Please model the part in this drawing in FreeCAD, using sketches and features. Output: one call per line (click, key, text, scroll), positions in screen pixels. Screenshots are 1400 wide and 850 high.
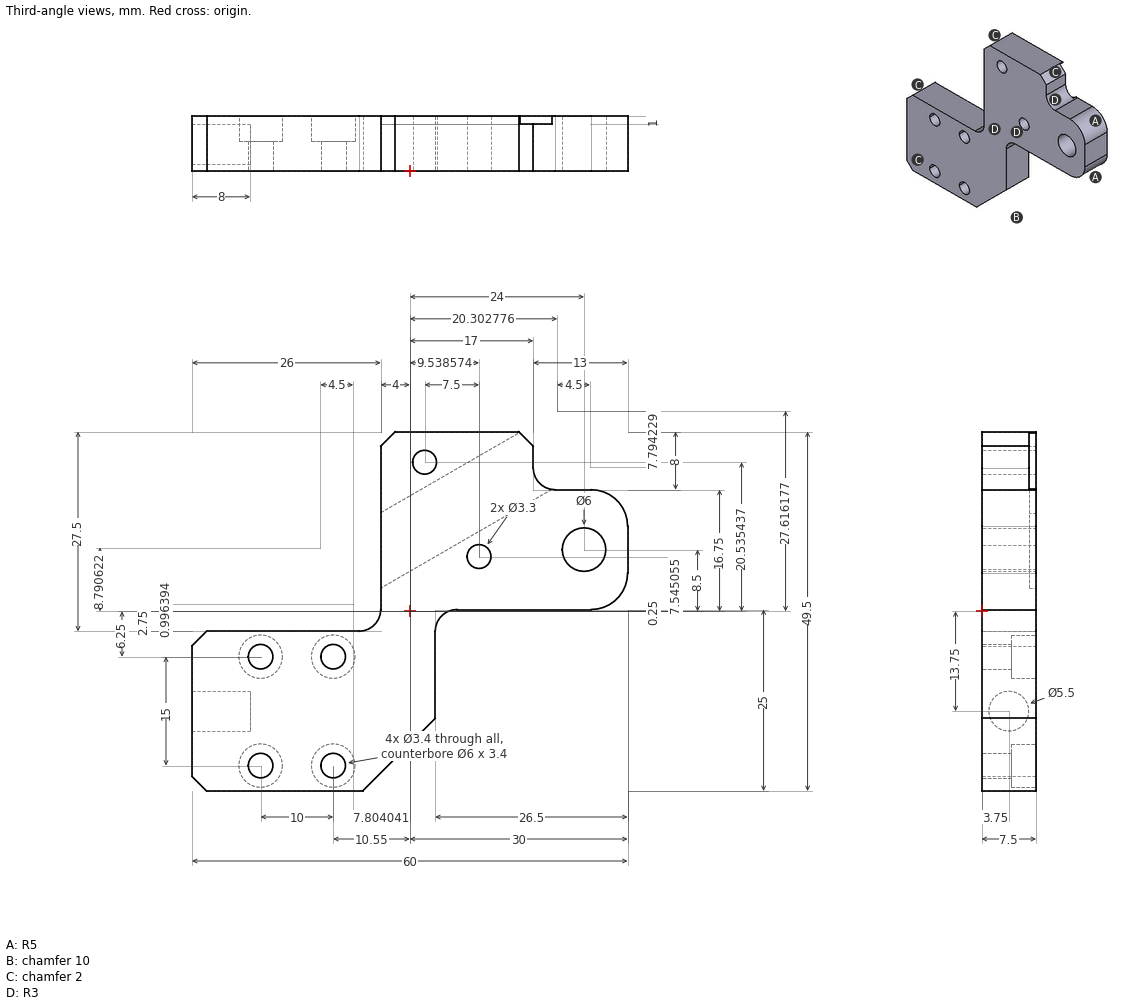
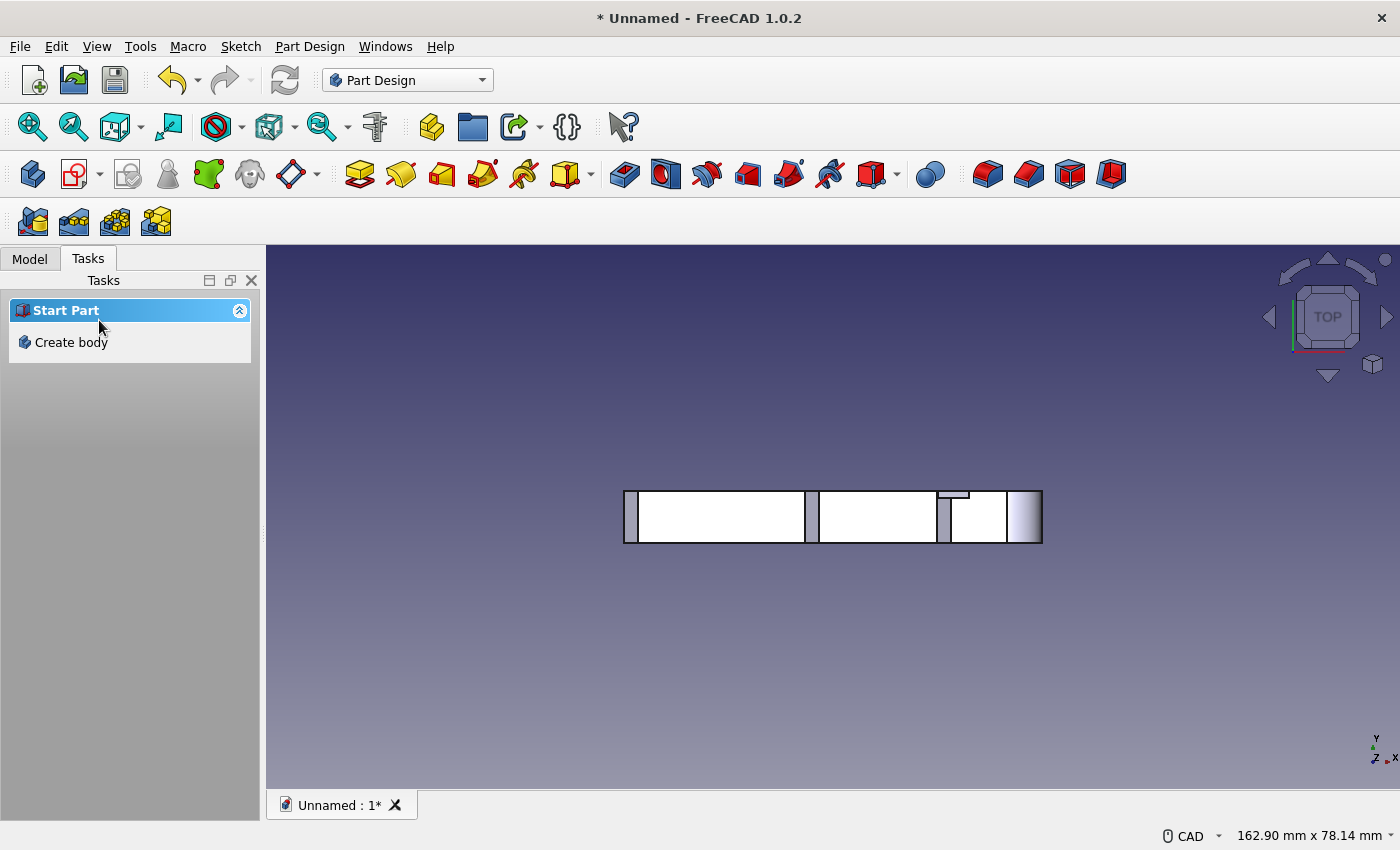
key(1)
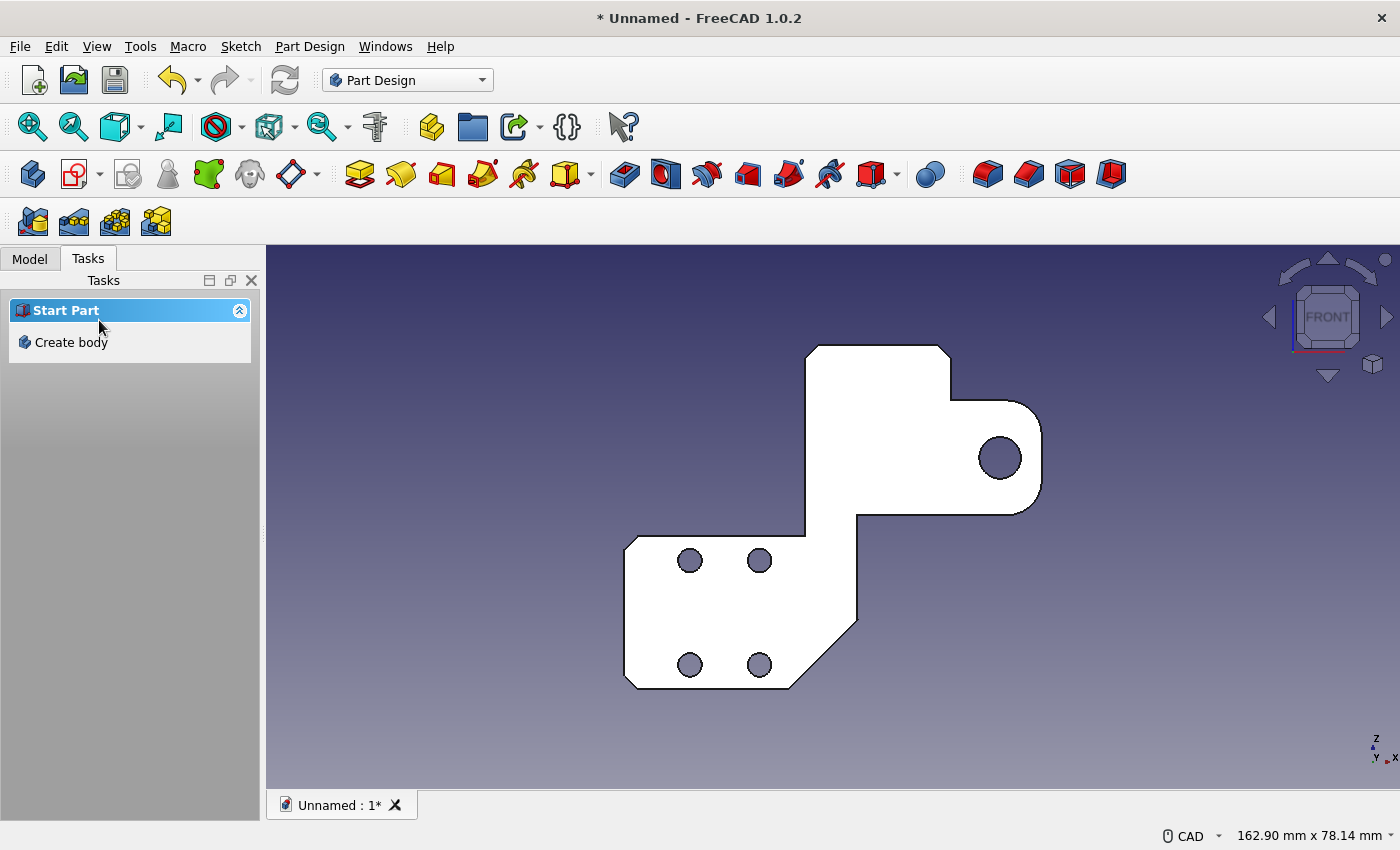
key(3)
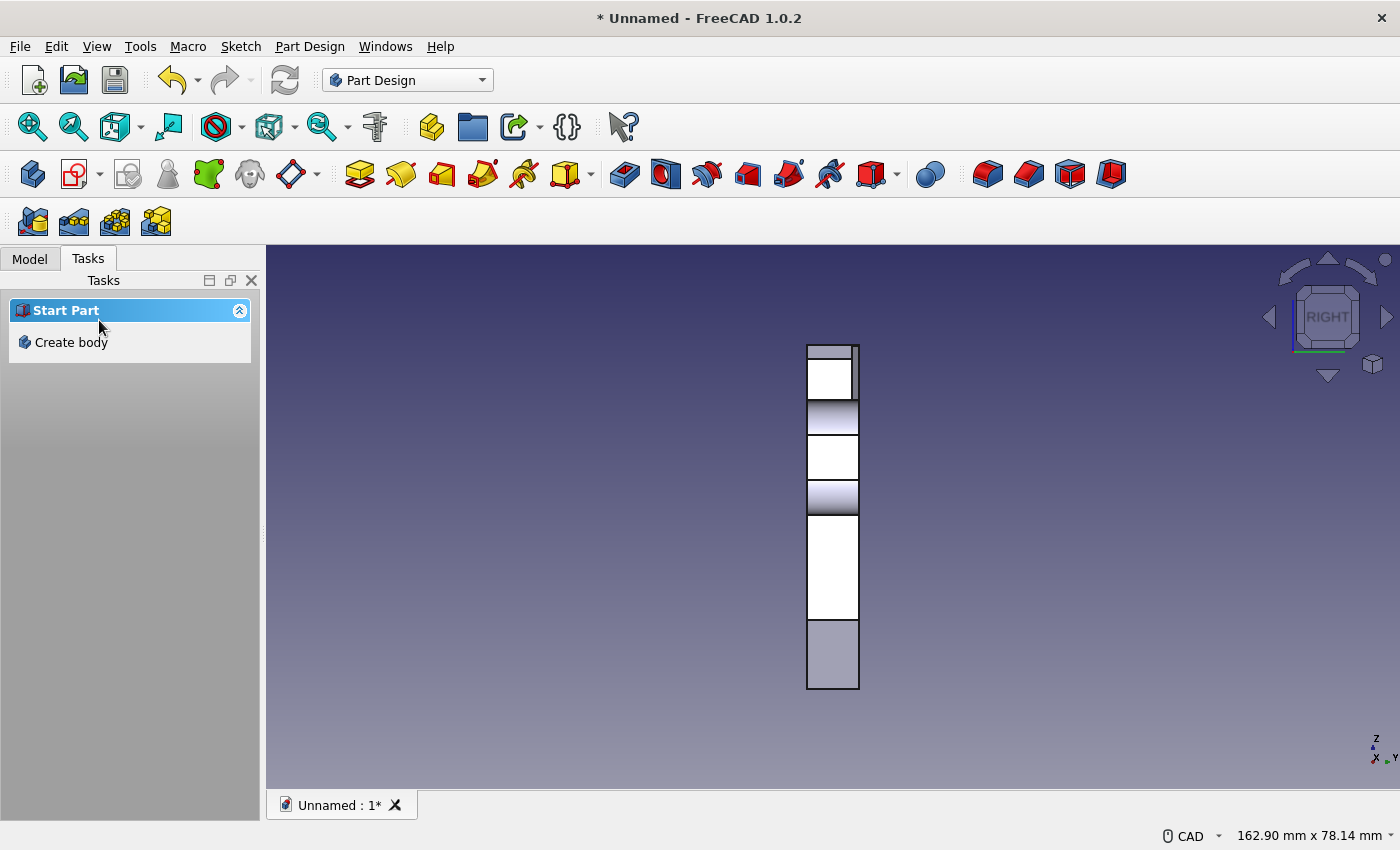
key(5)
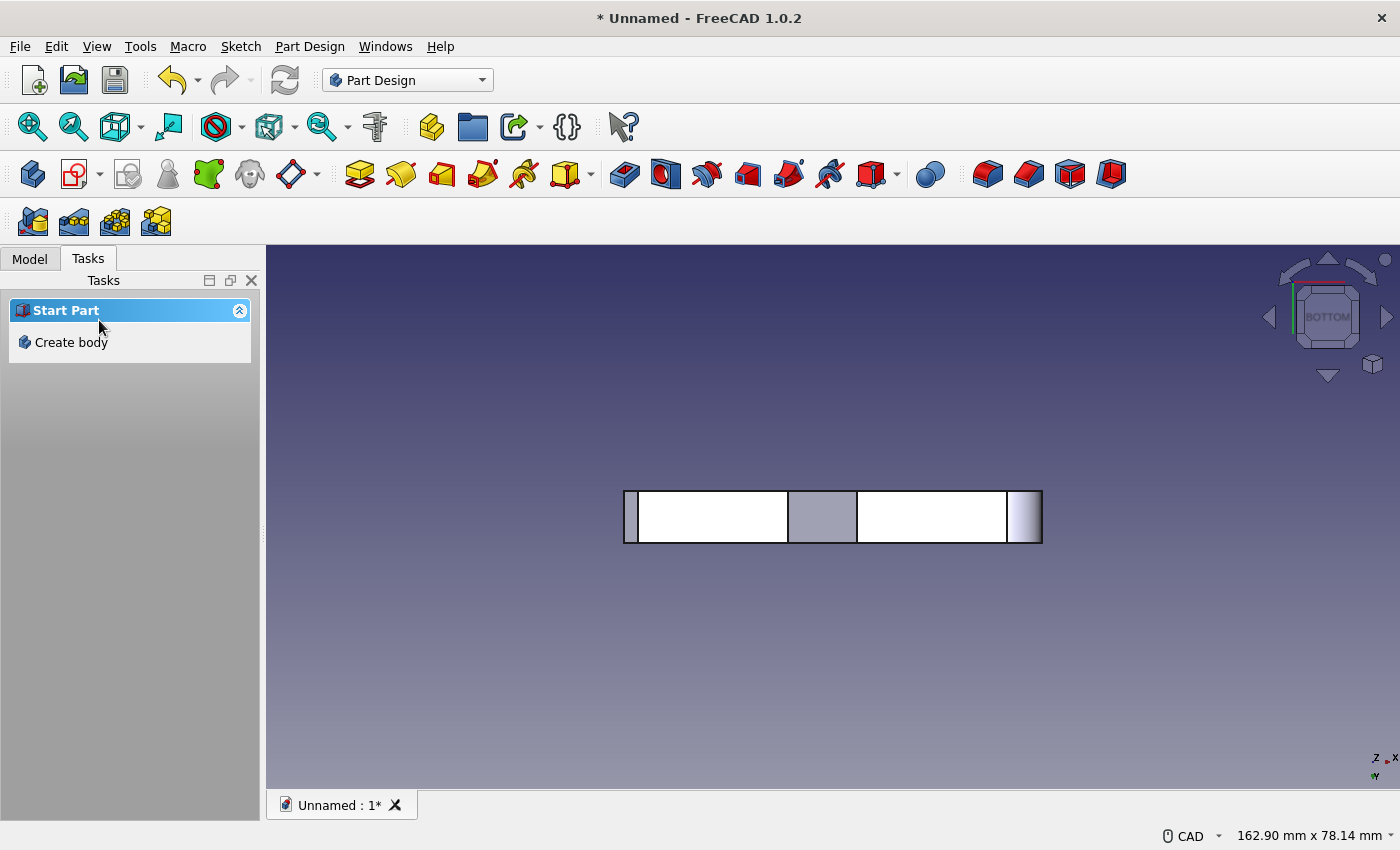
key(v)
key(f)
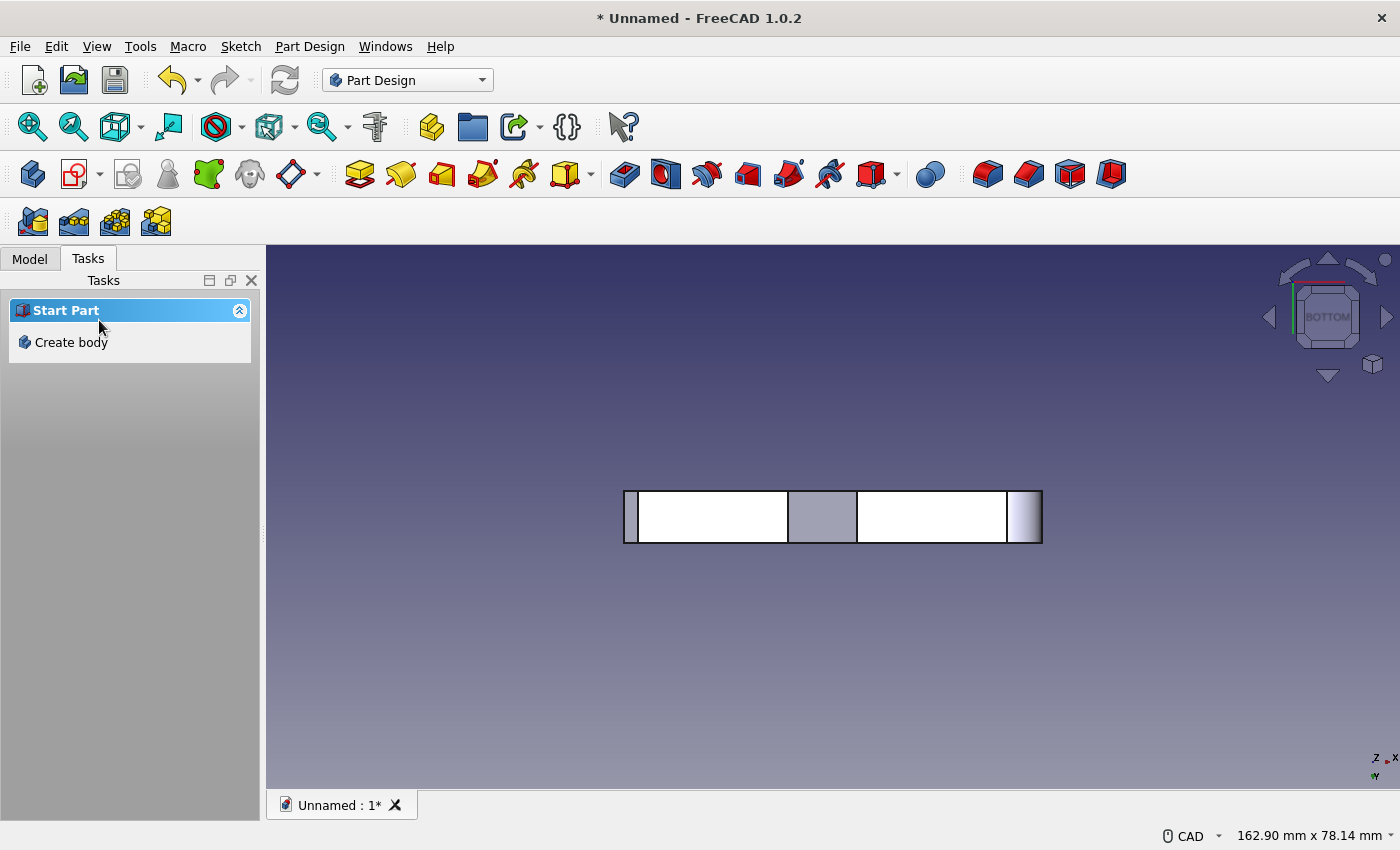
key(4)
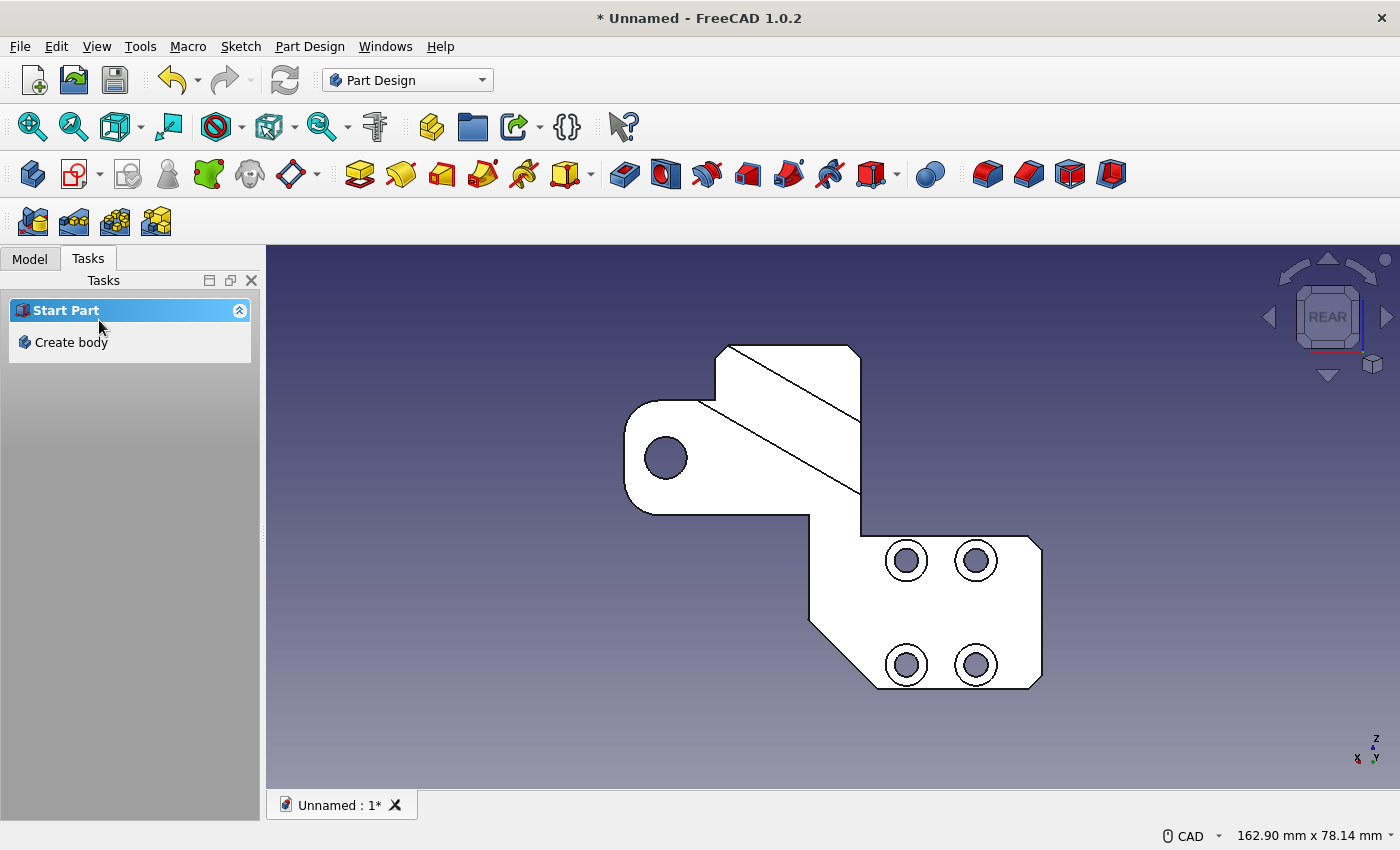
key(6)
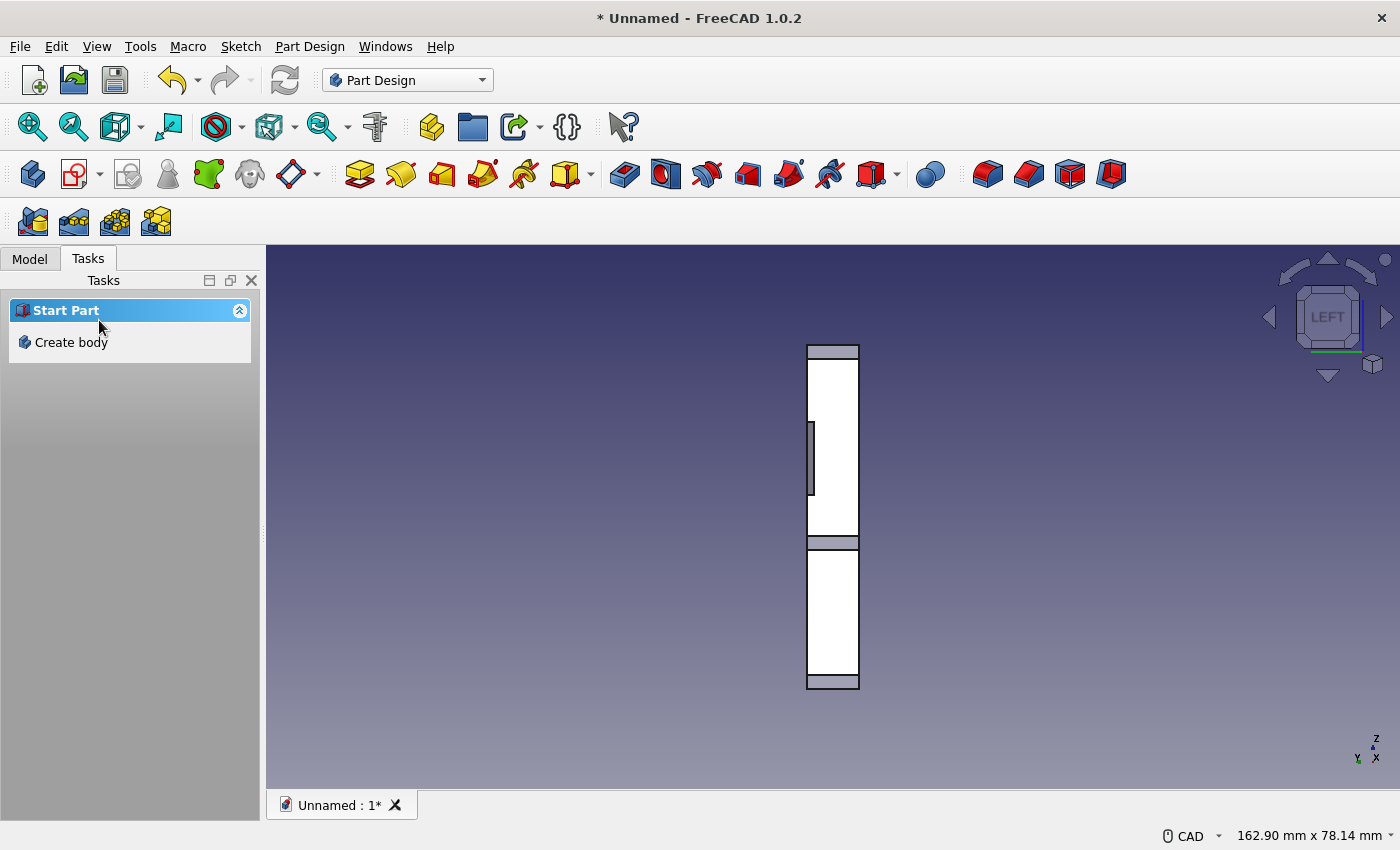
key(v)
key(3)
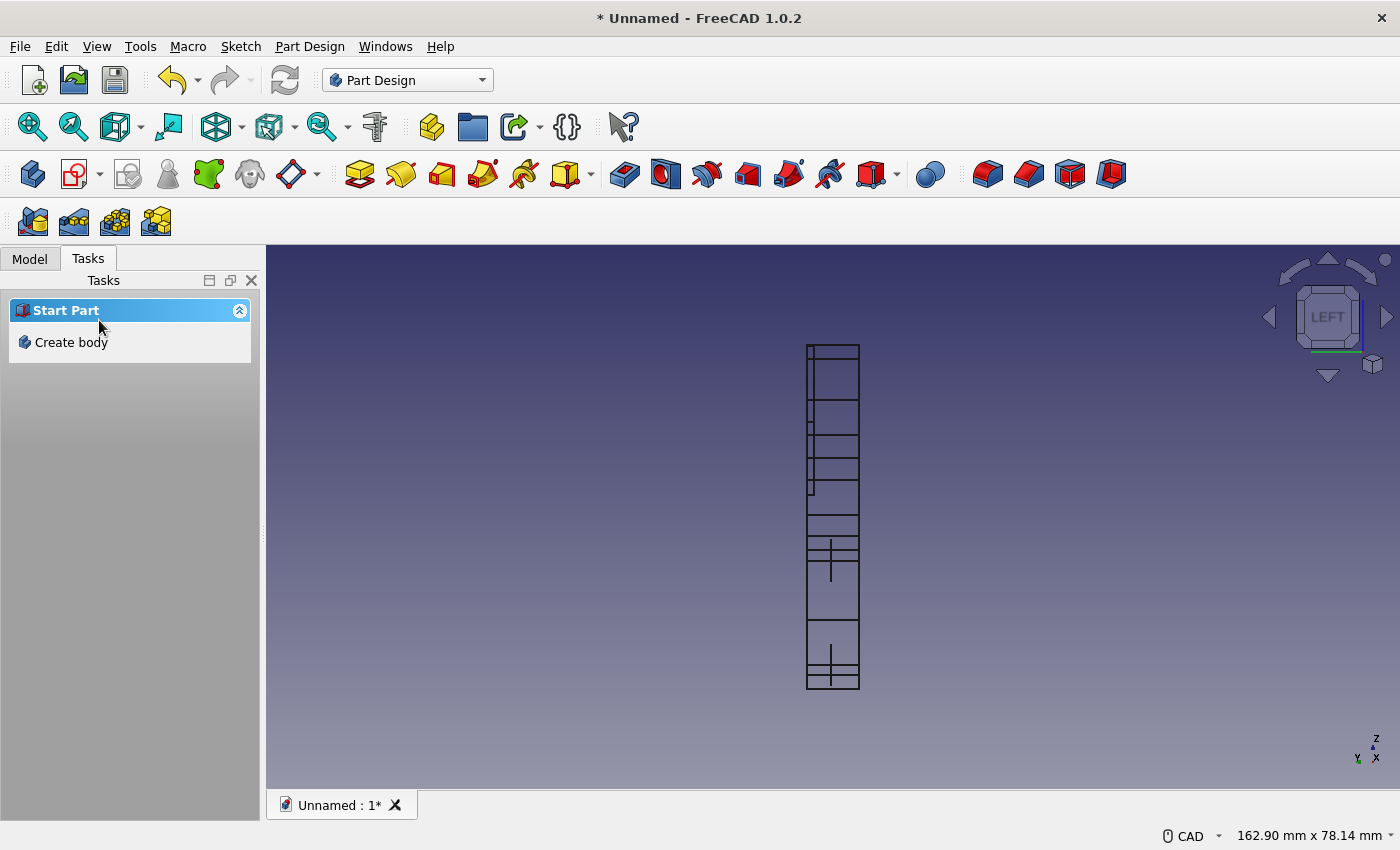
key(0)